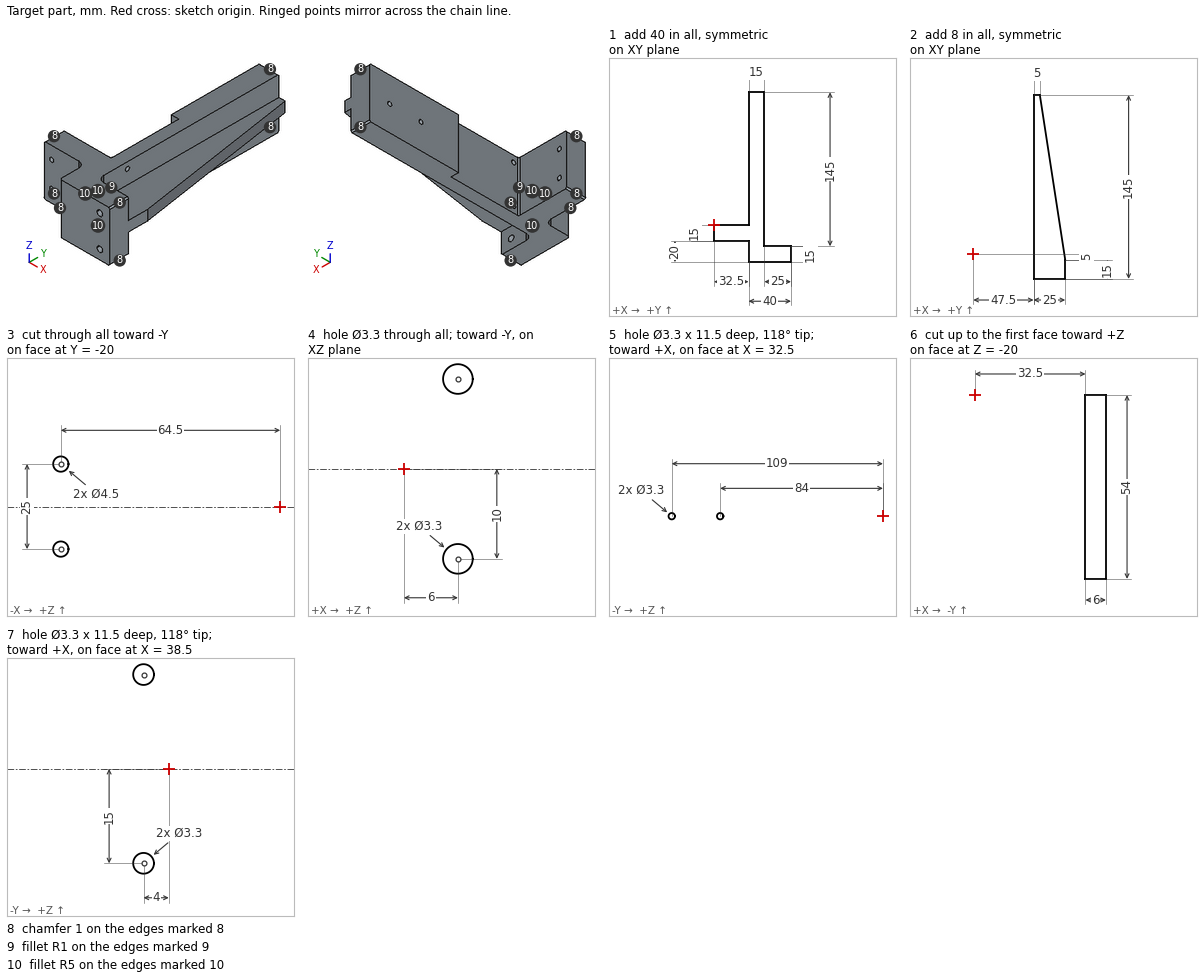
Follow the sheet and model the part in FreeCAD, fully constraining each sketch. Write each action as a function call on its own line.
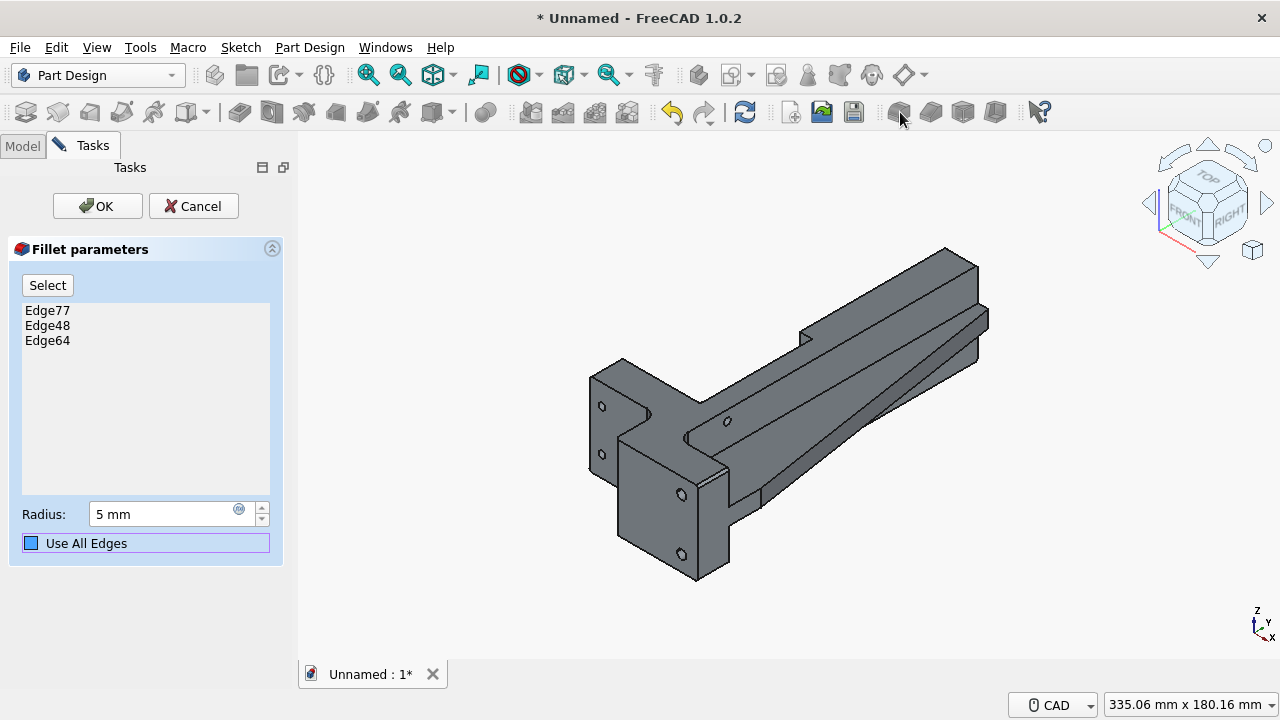
click(98, 206)